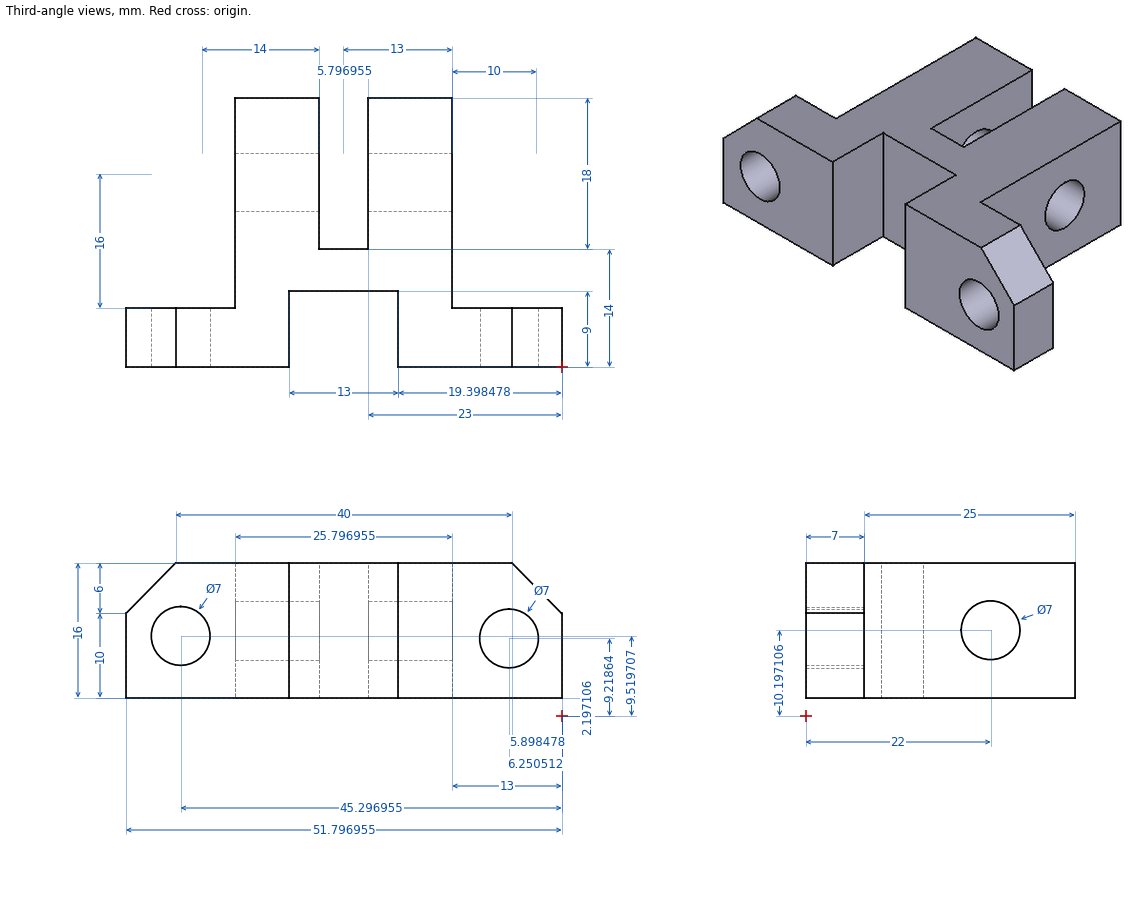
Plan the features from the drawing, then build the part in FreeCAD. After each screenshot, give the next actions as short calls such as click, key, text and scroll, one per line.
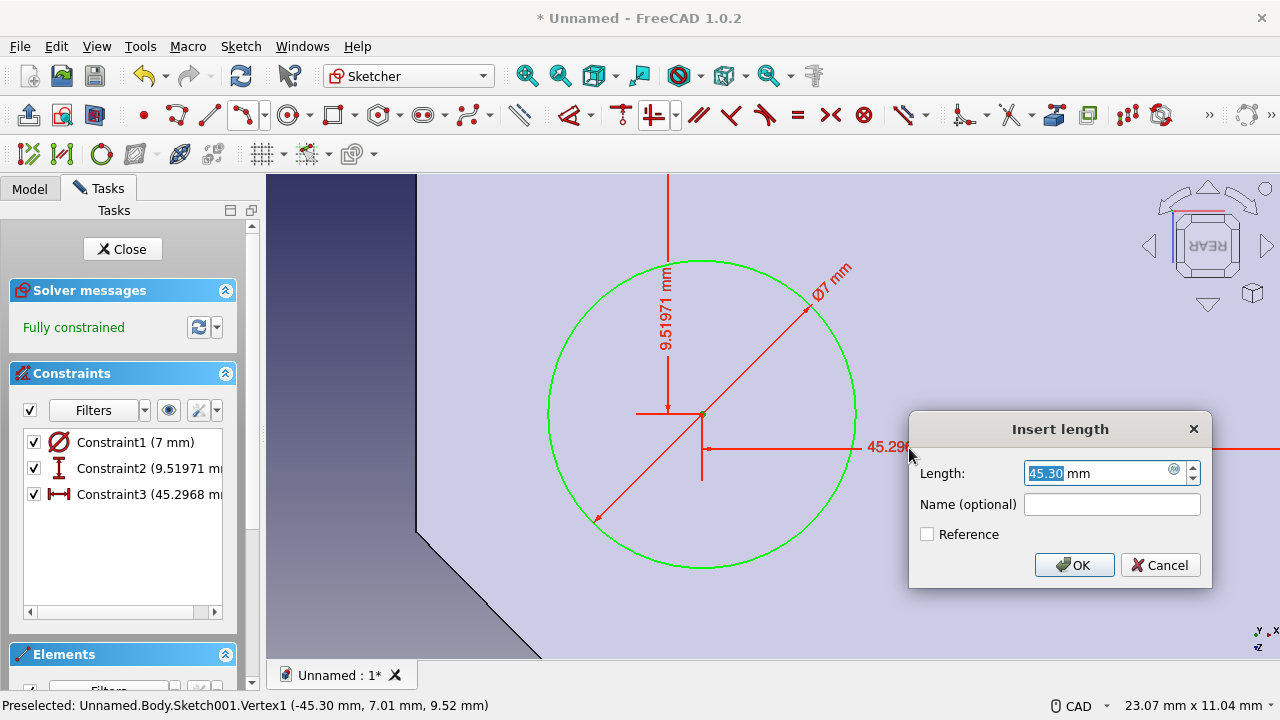
text(45.296955)
key(Return)
key(Escape)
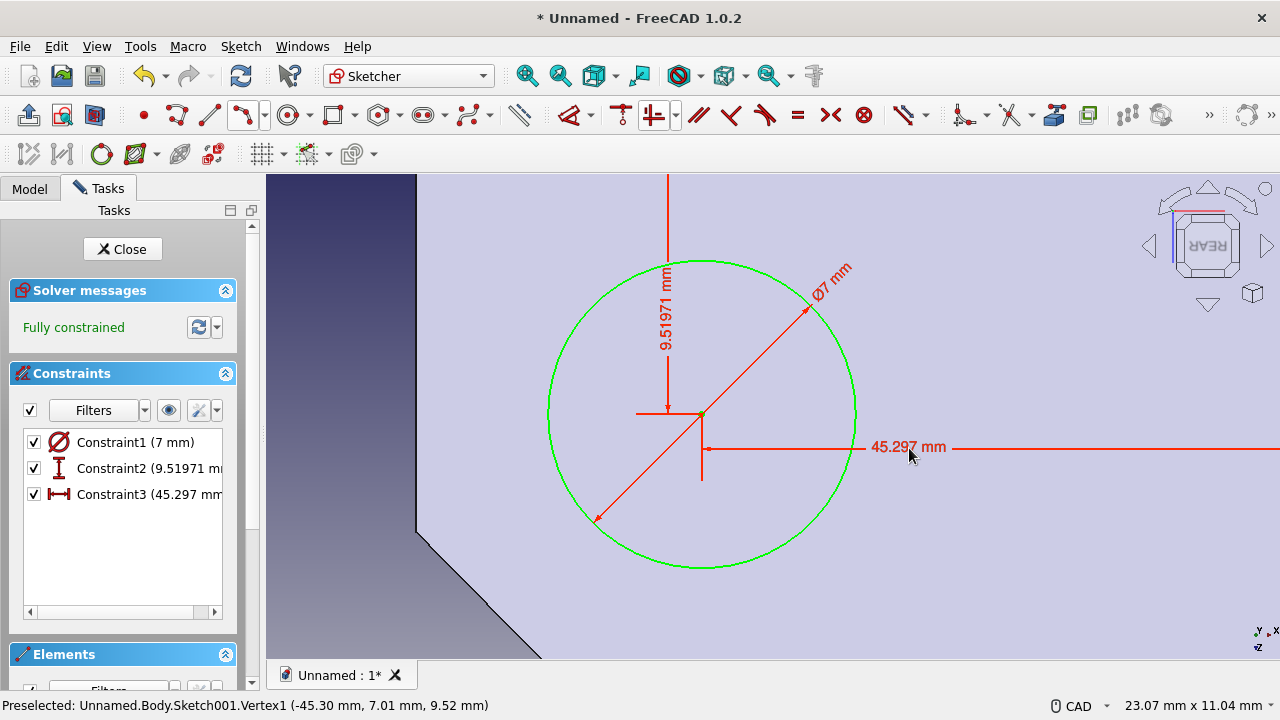
click(123, 249)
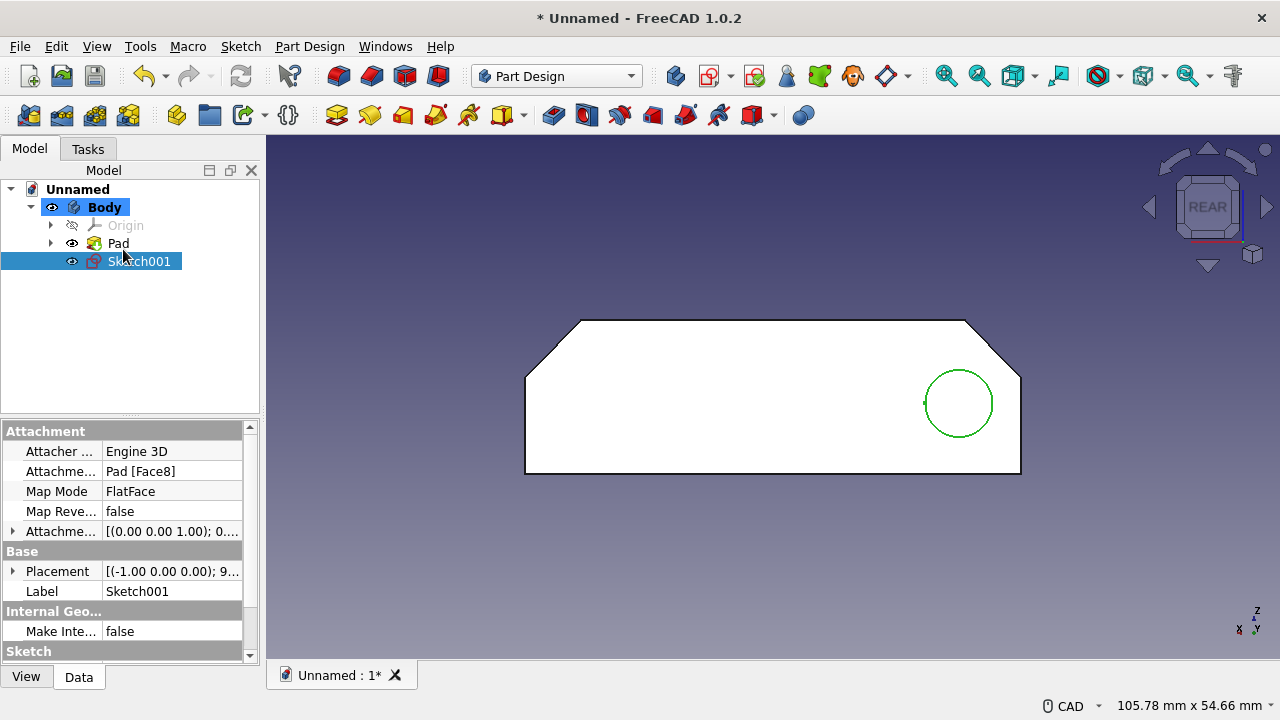
click(554, 116)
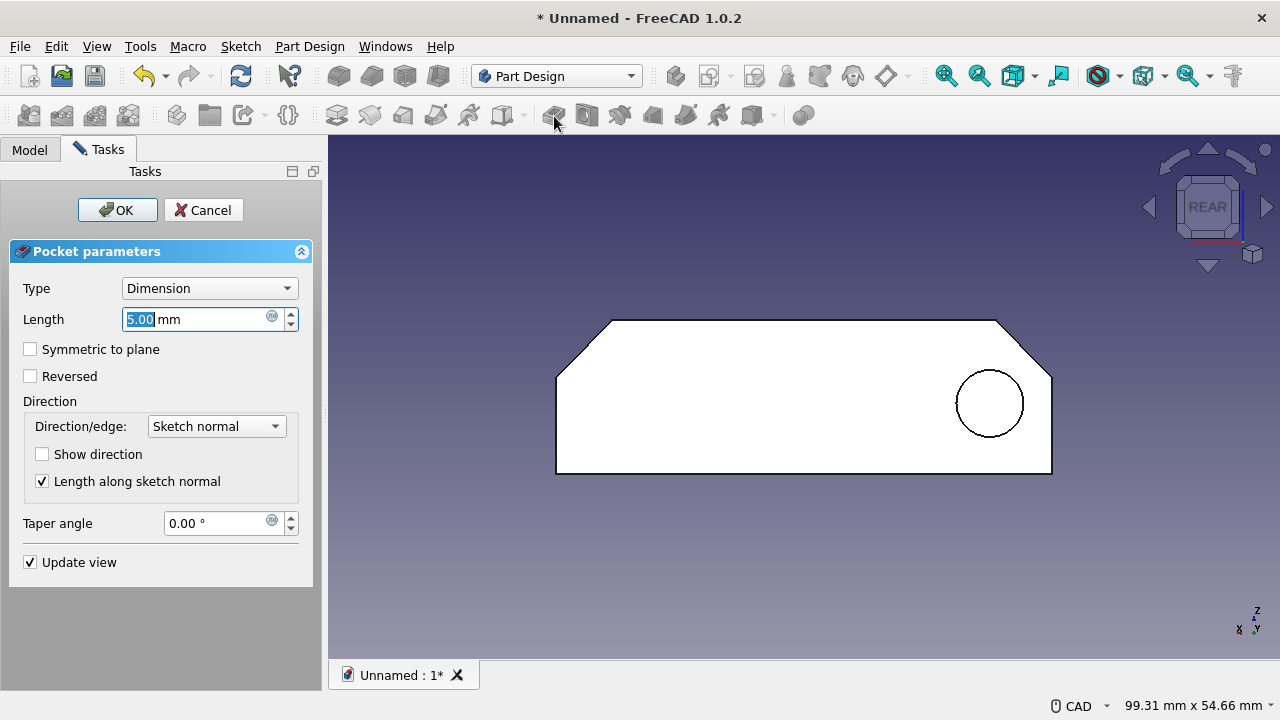
click(210, 288)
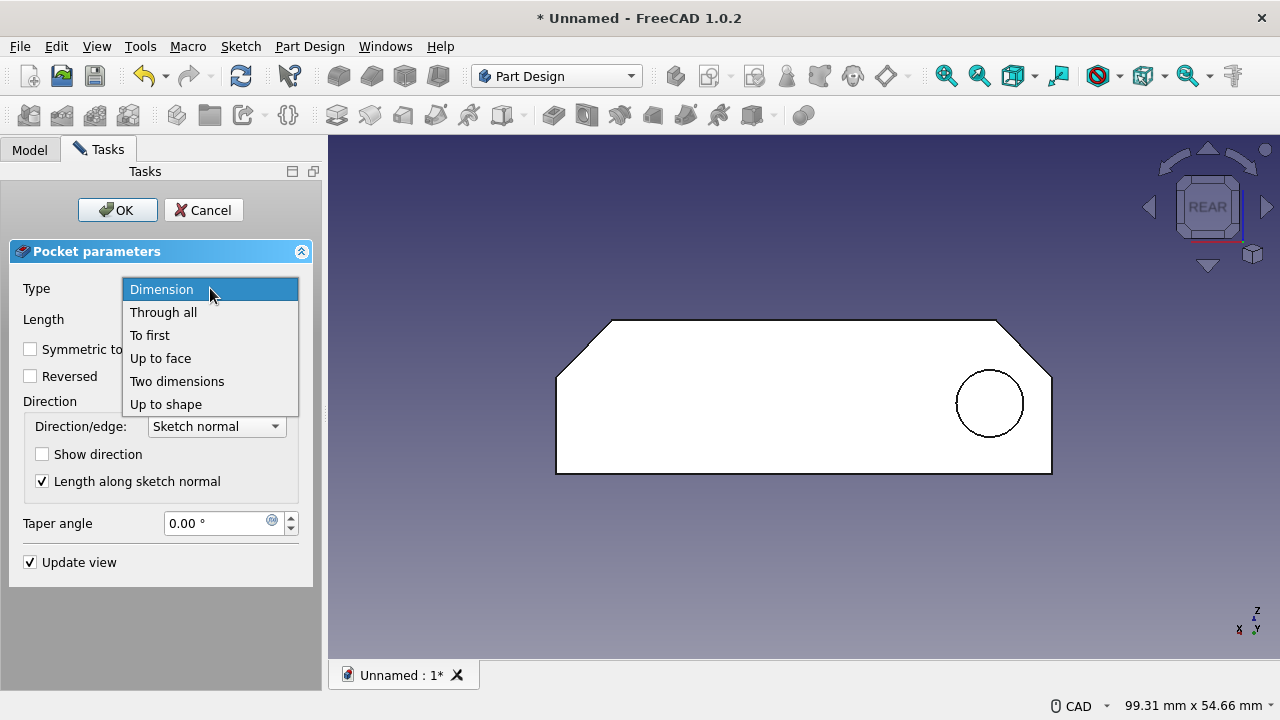
click(208, 382)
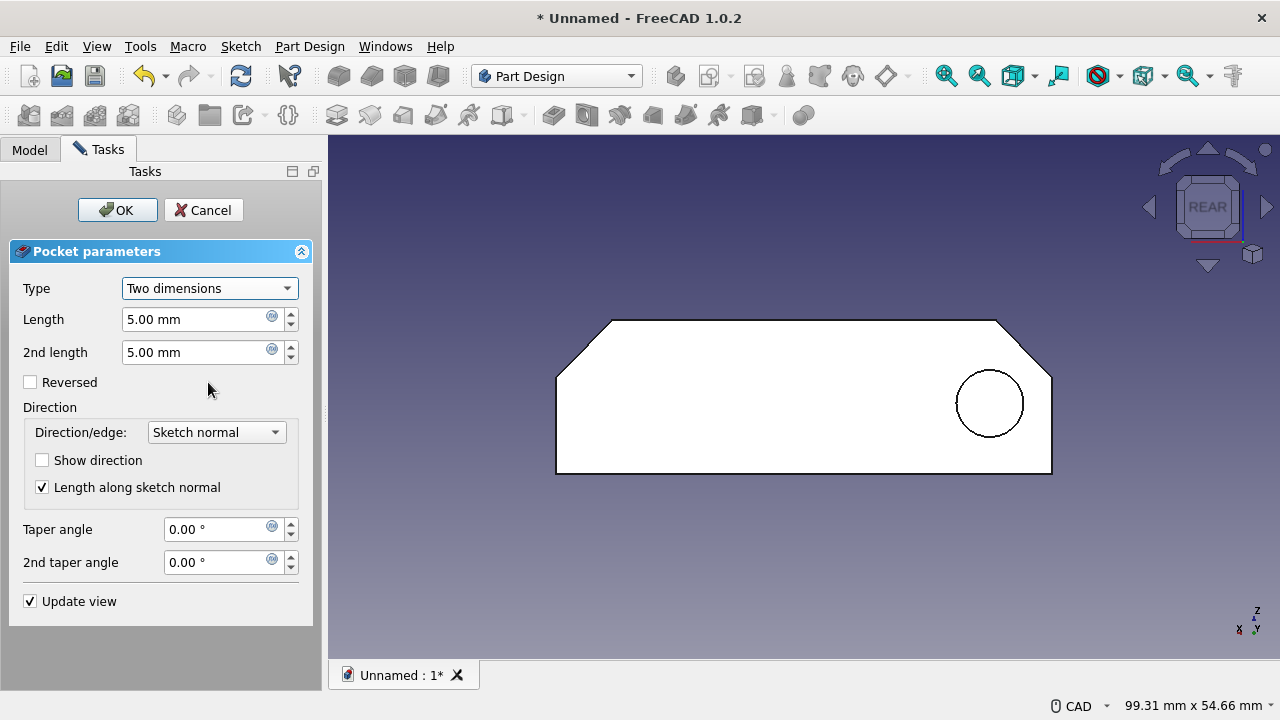
triple_click(204, 320)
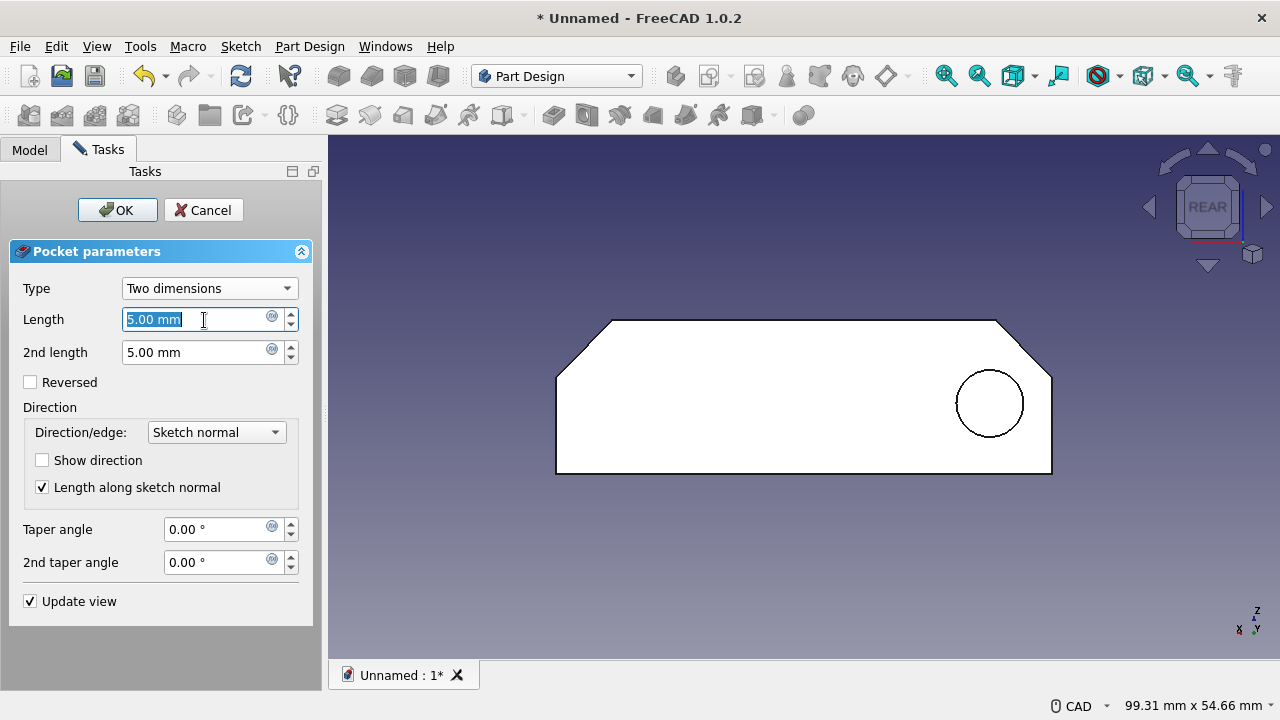
text(16)
key(Tab)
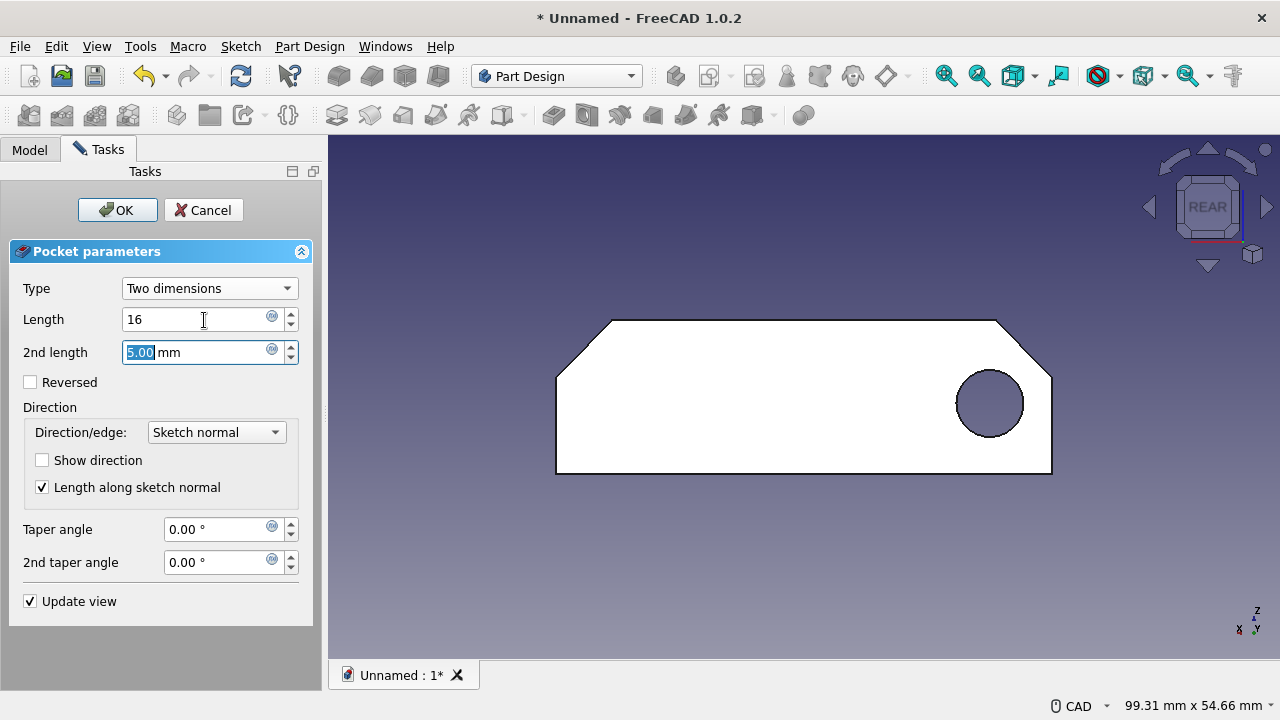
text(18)
key(Tab)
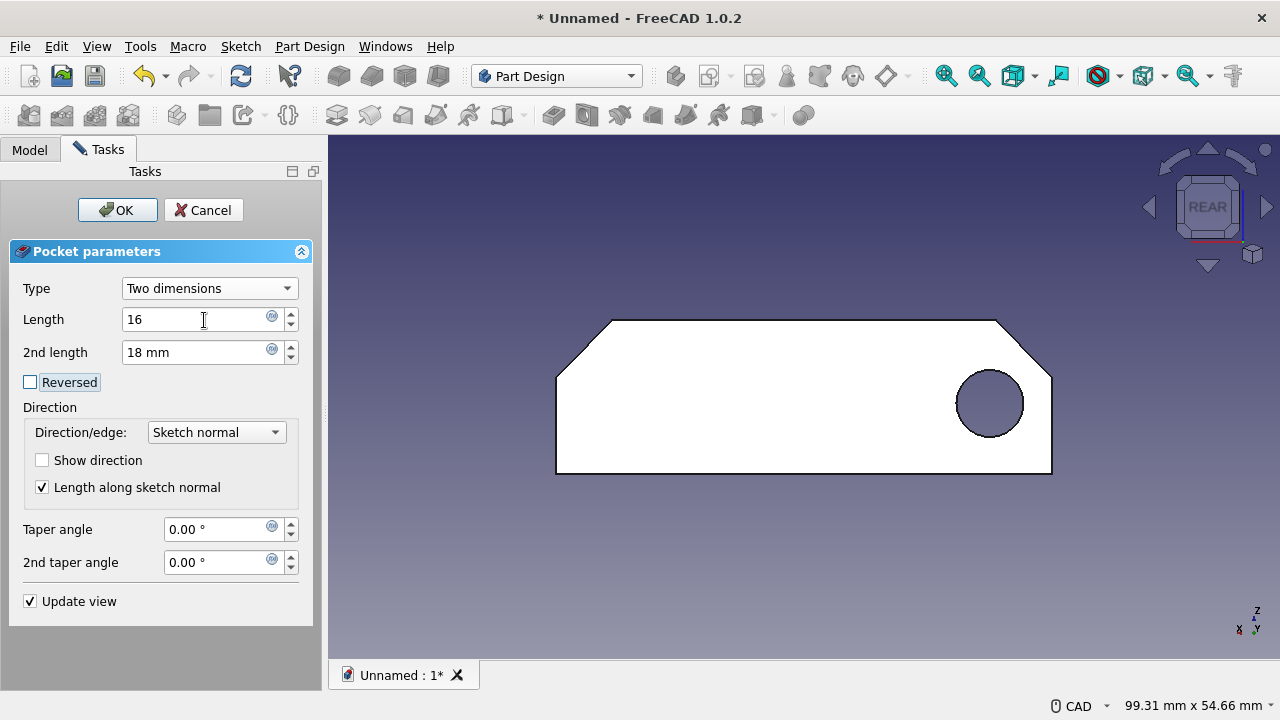
click(31, 382)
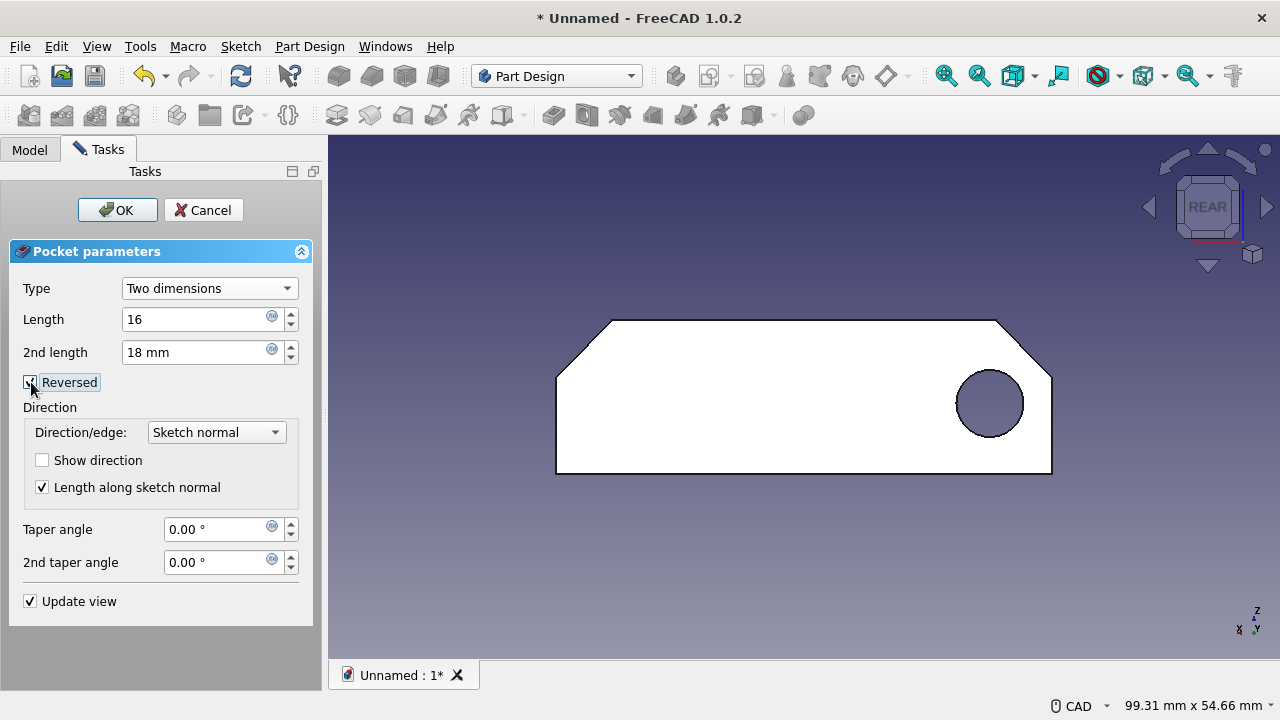
click(118, 210)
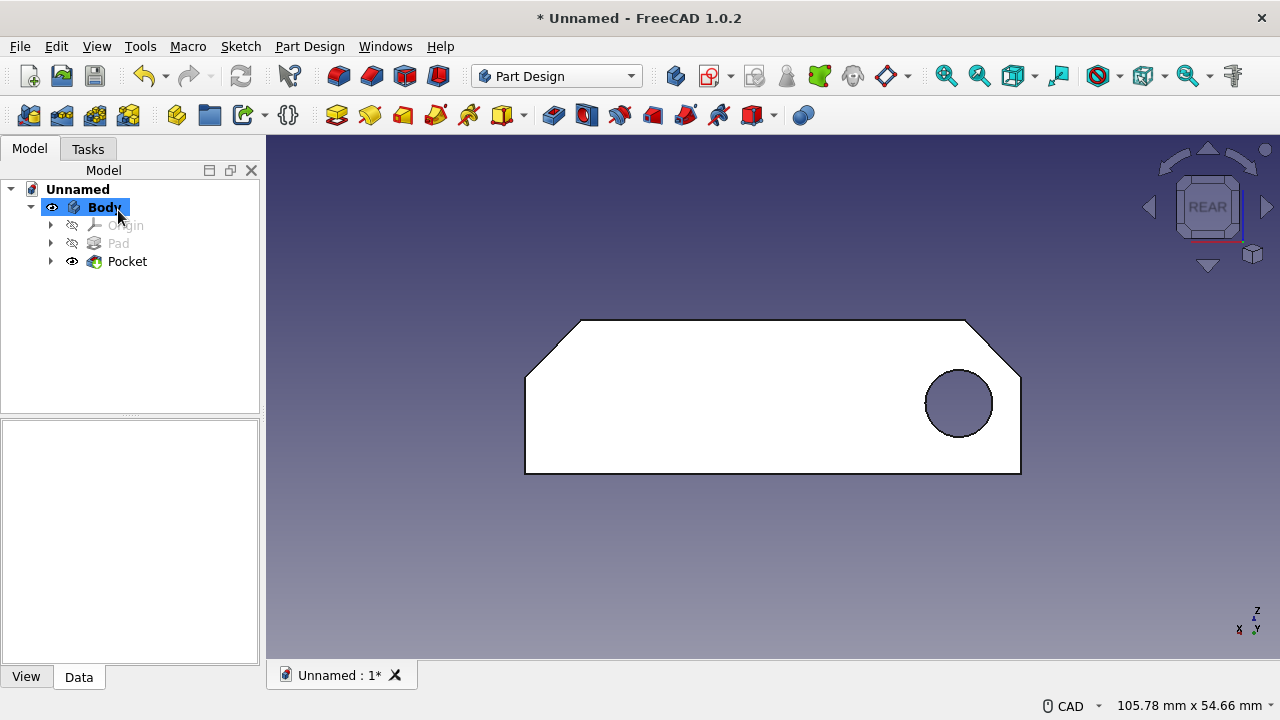
click(631, 396)